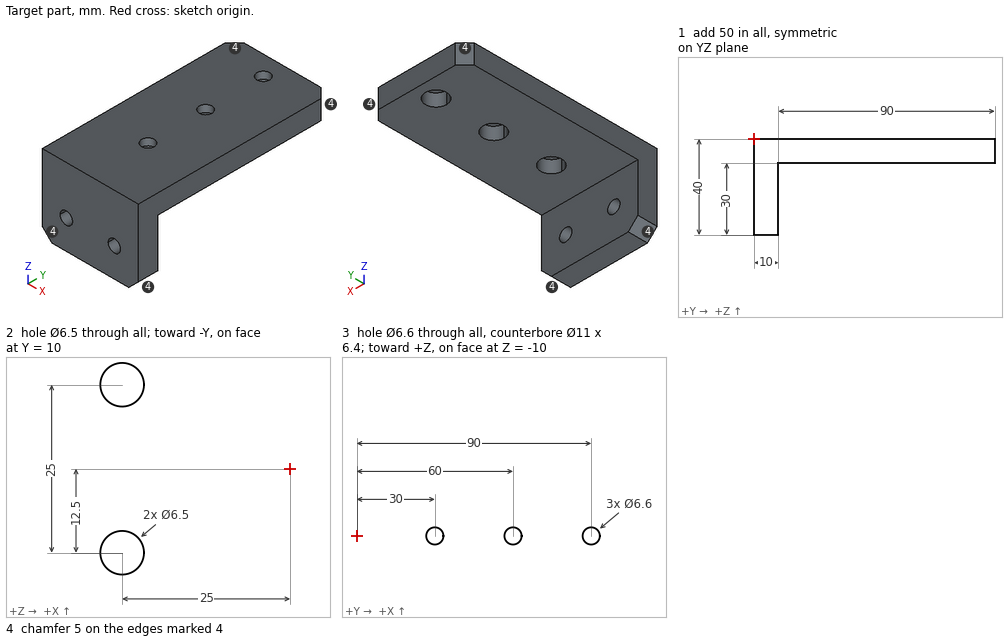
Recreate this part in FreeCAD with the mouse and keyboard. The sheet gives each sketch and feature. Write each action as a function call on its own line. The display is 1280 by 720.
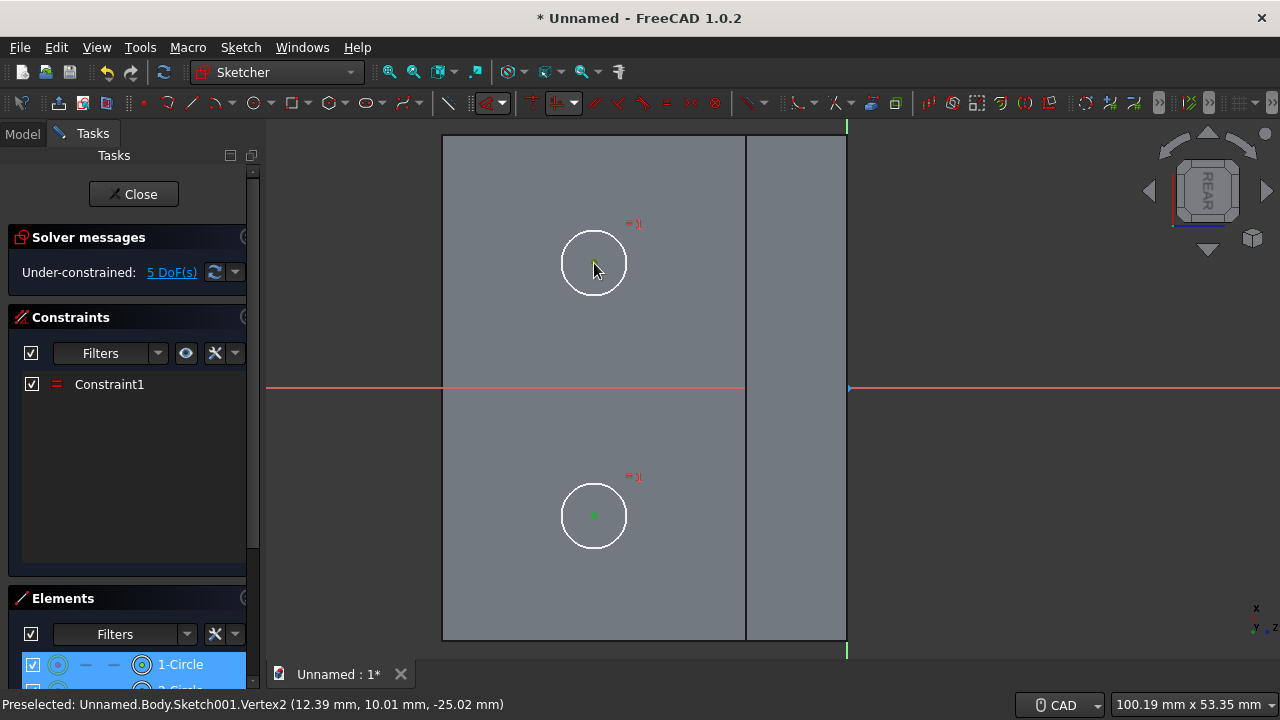
click(576, 104)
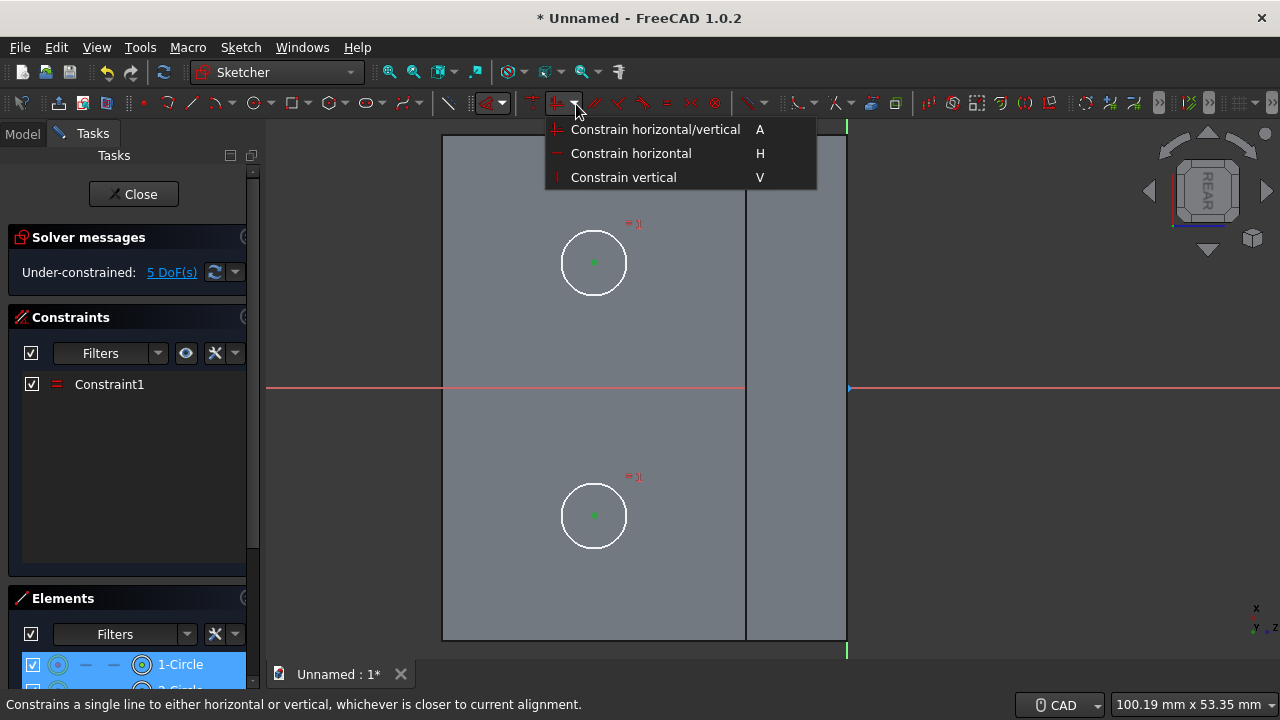
click(681, 177)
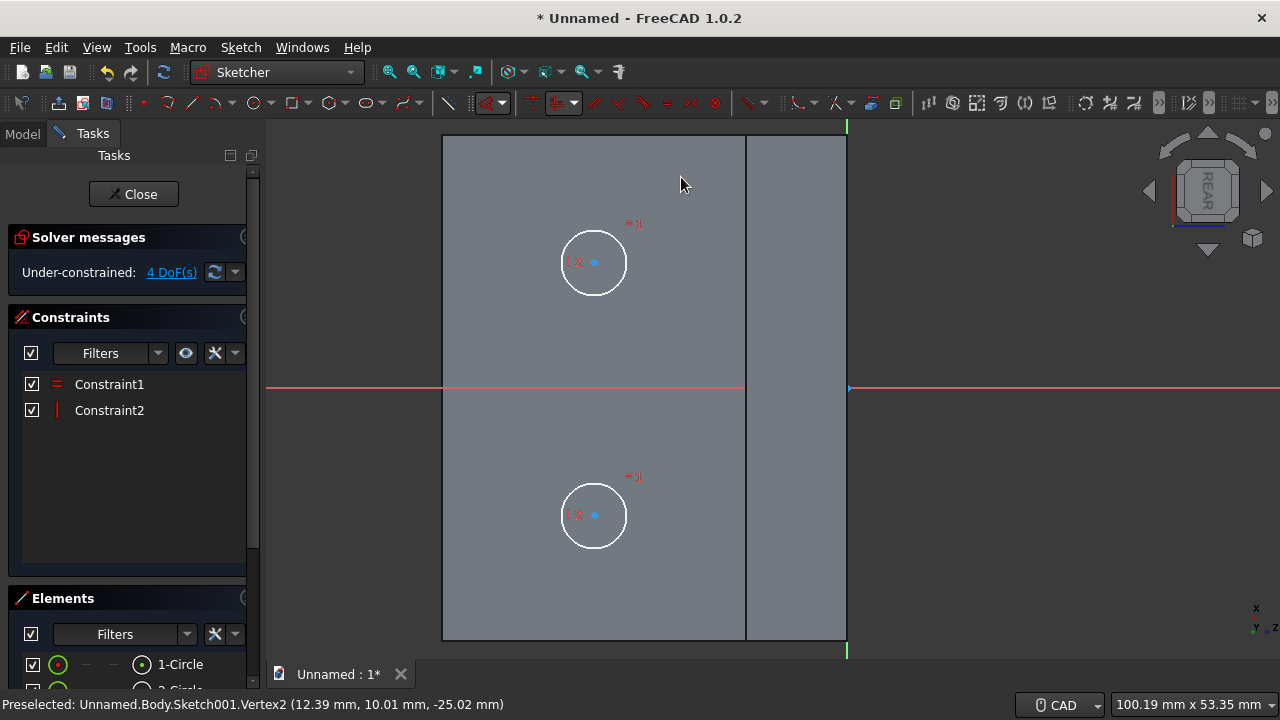
click(617, 493)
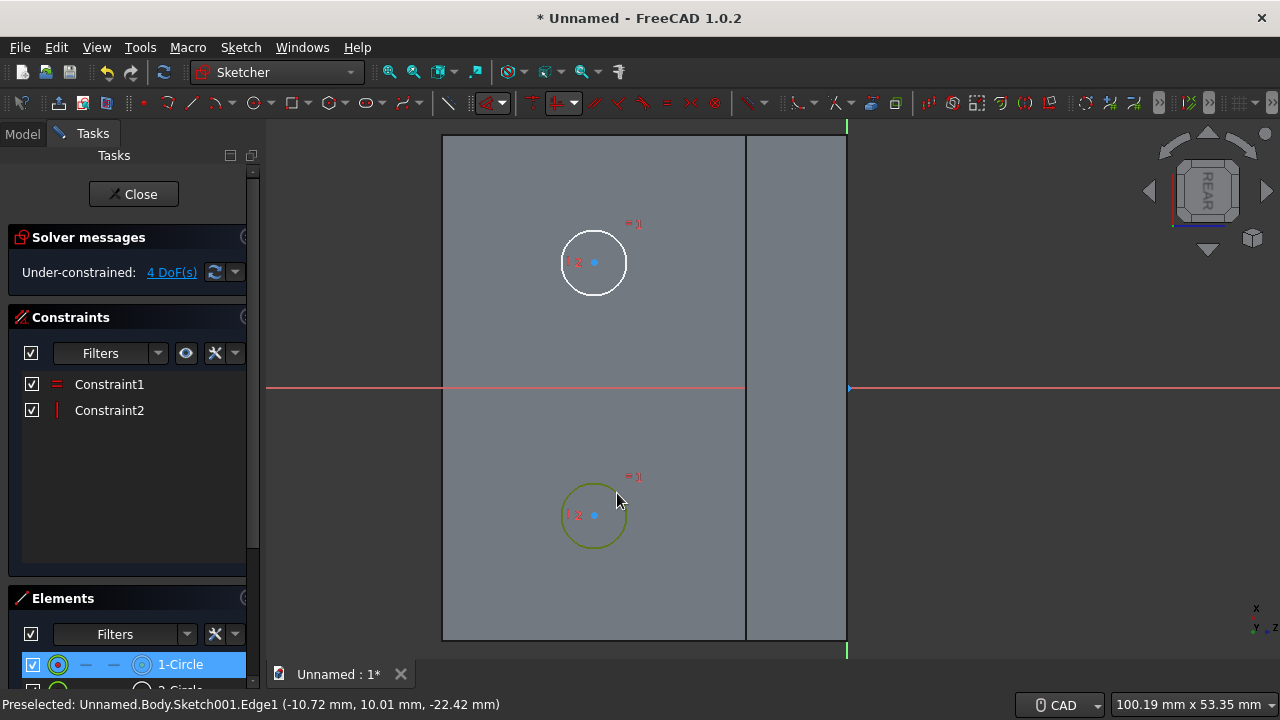
key(k)
key(o)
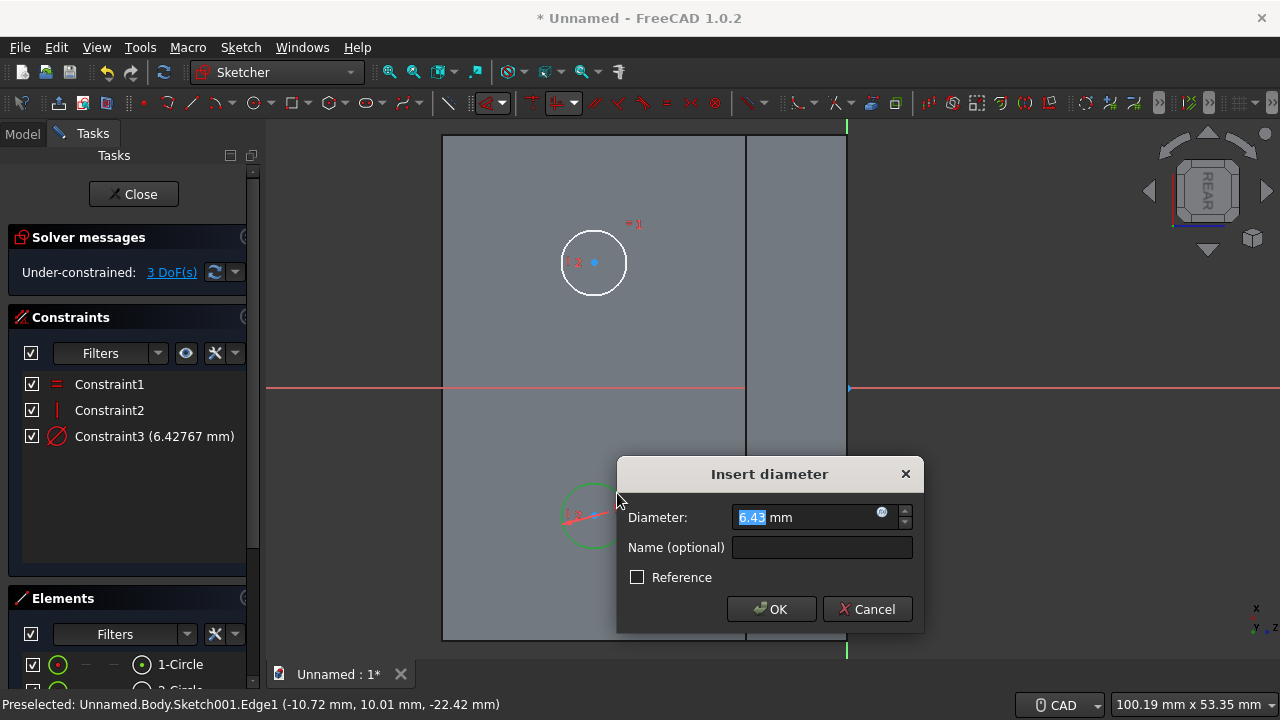
text(6.5)
key(Return)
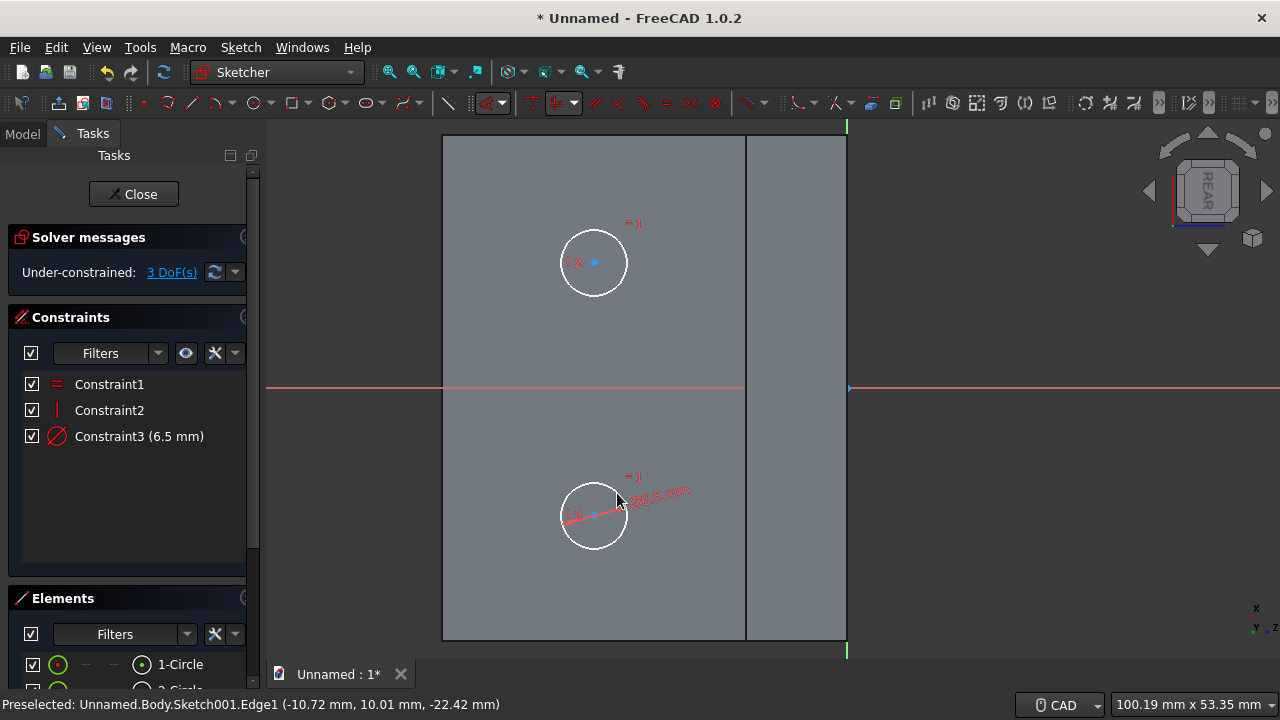
click(594, 516)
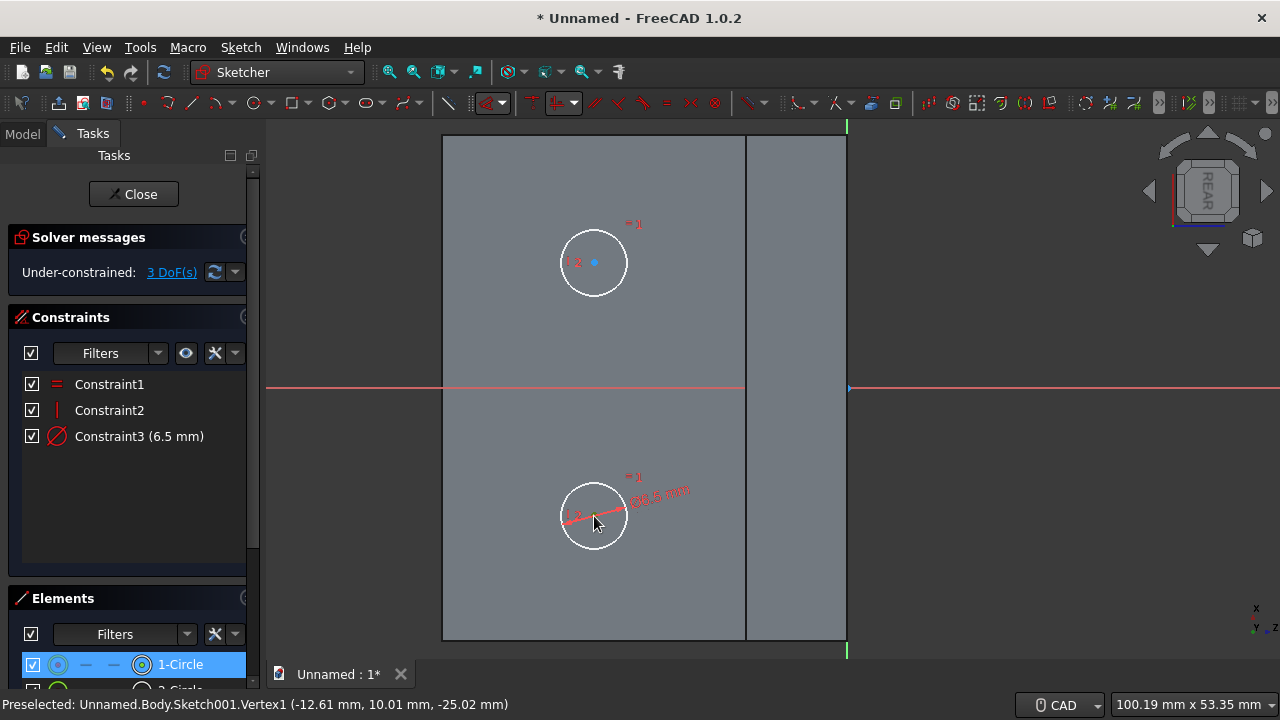
click(504, 104)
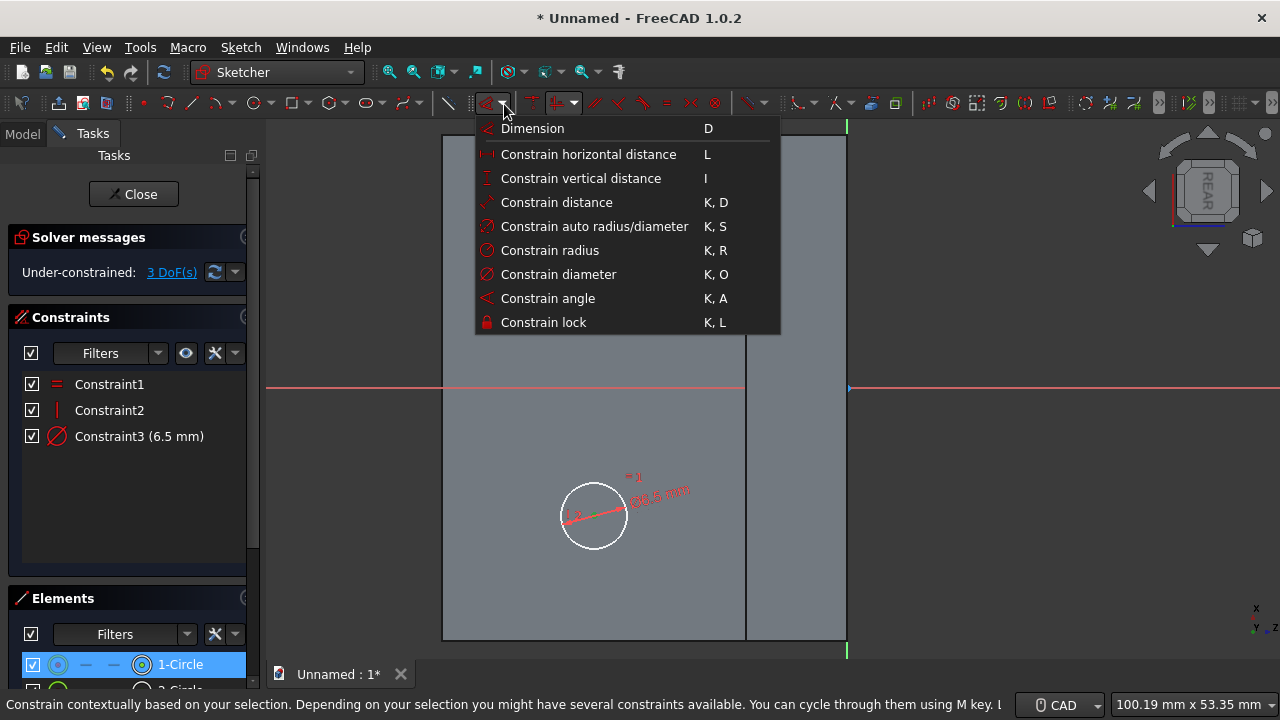
click(628, 154)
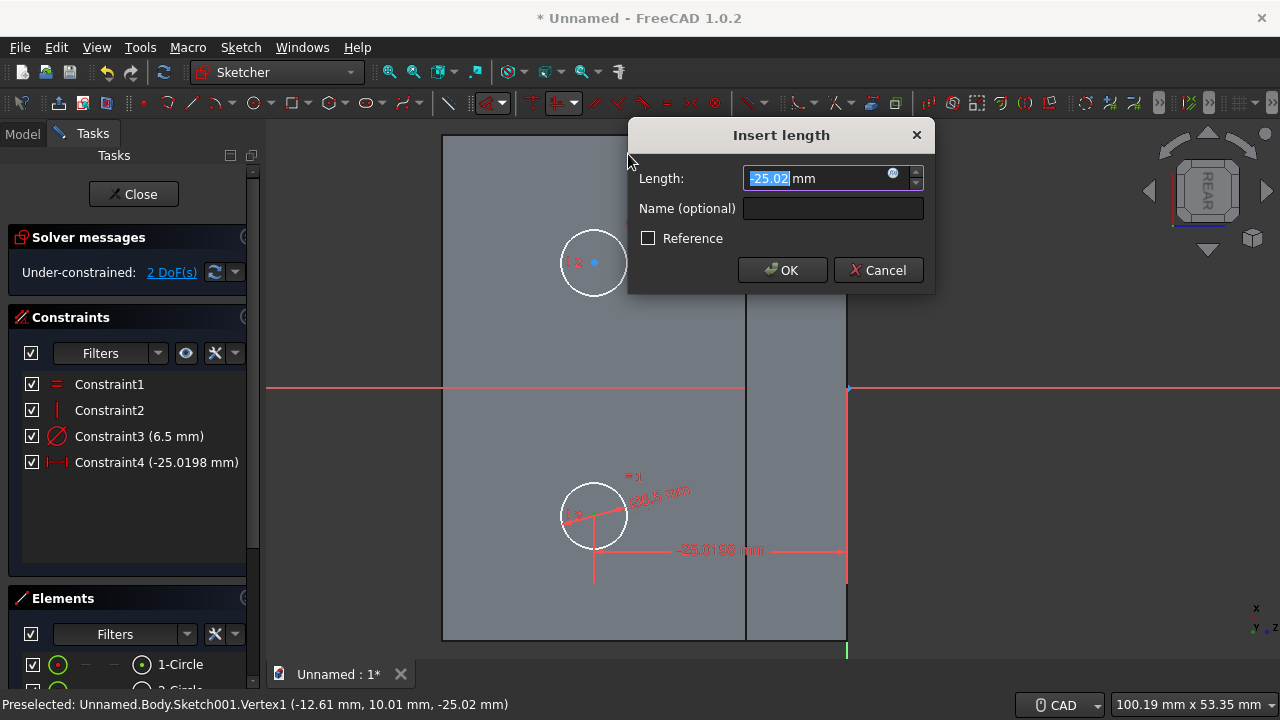
text(-25)
key(Return)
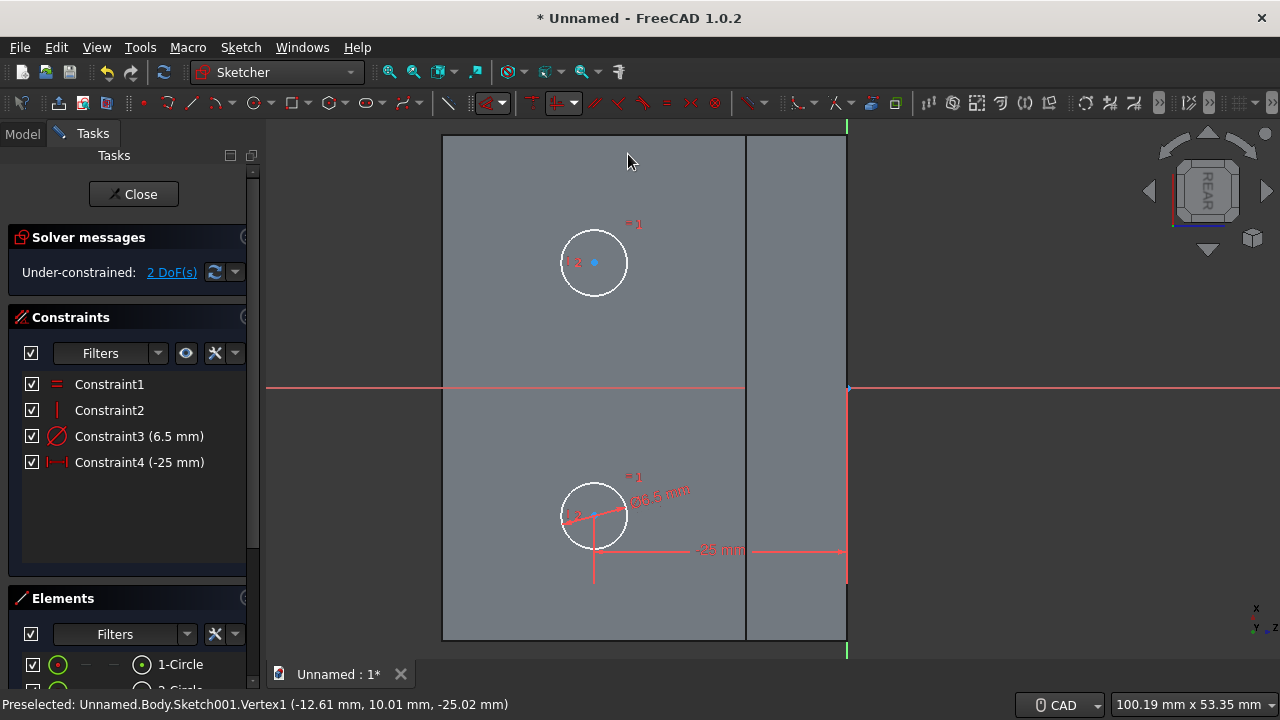
click(594, 516)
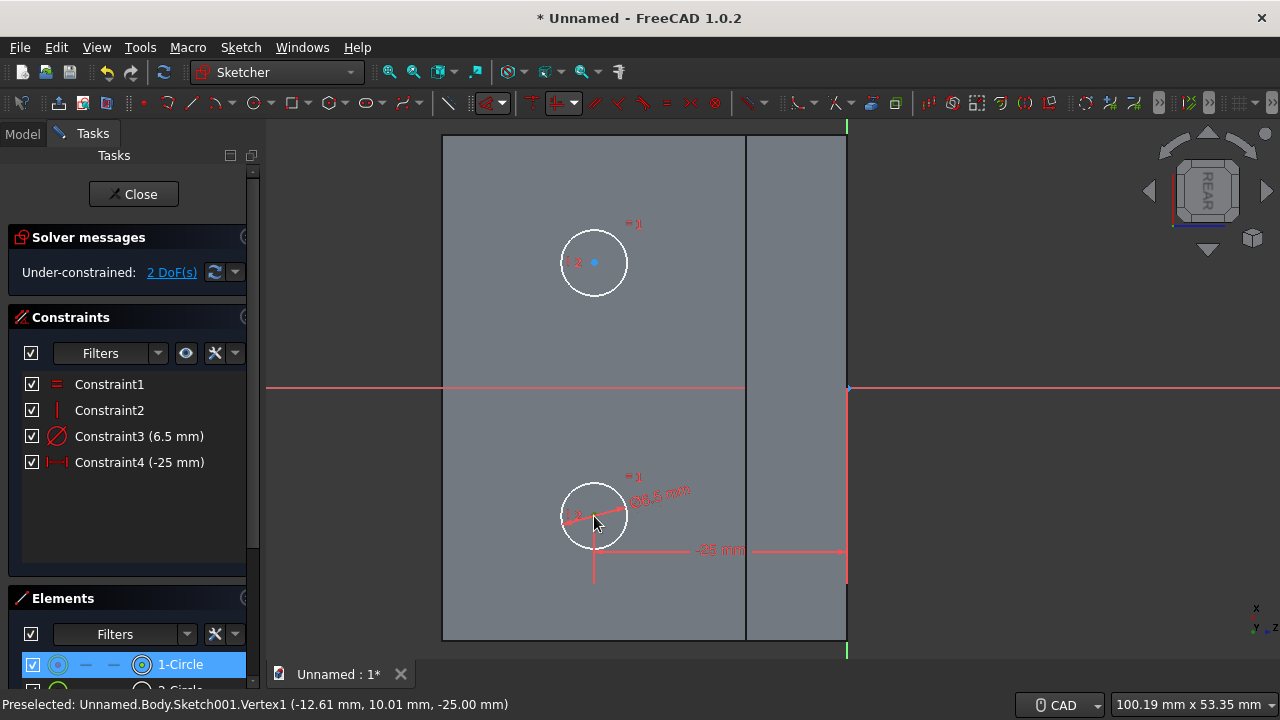
click(594, 263)